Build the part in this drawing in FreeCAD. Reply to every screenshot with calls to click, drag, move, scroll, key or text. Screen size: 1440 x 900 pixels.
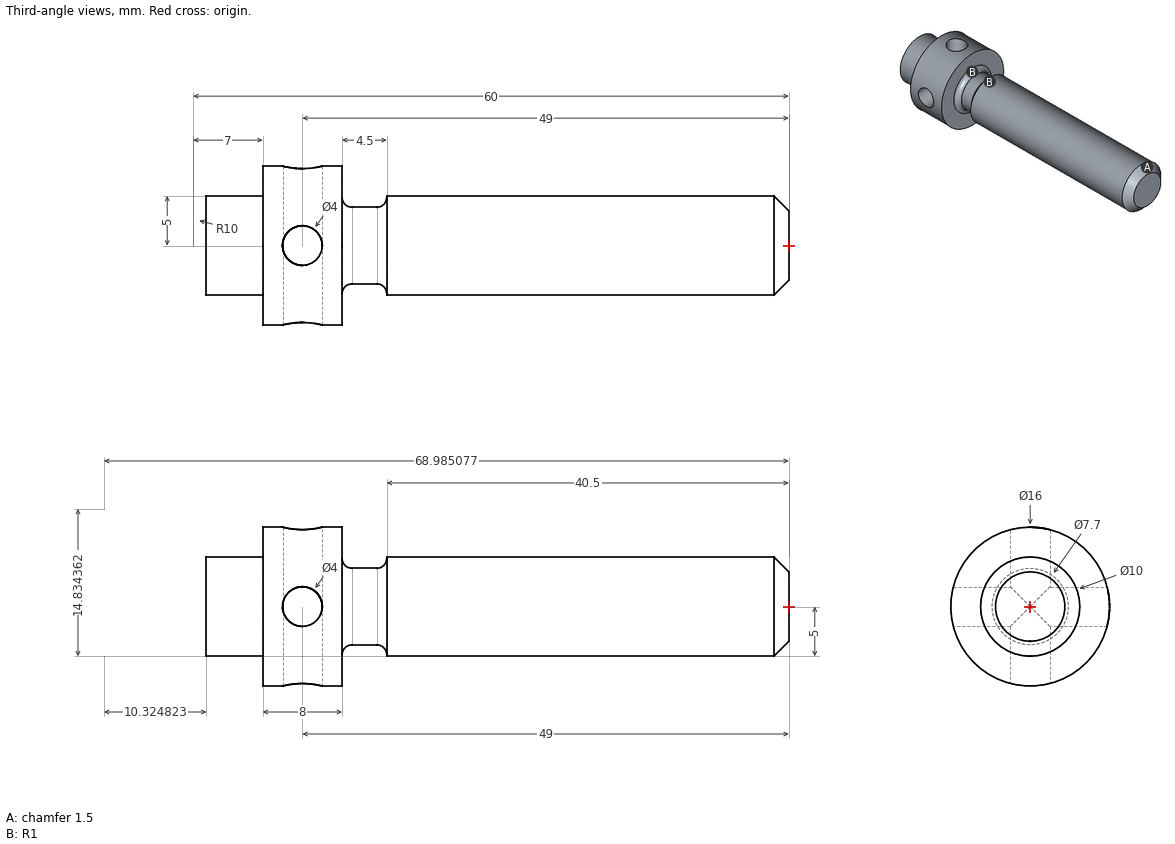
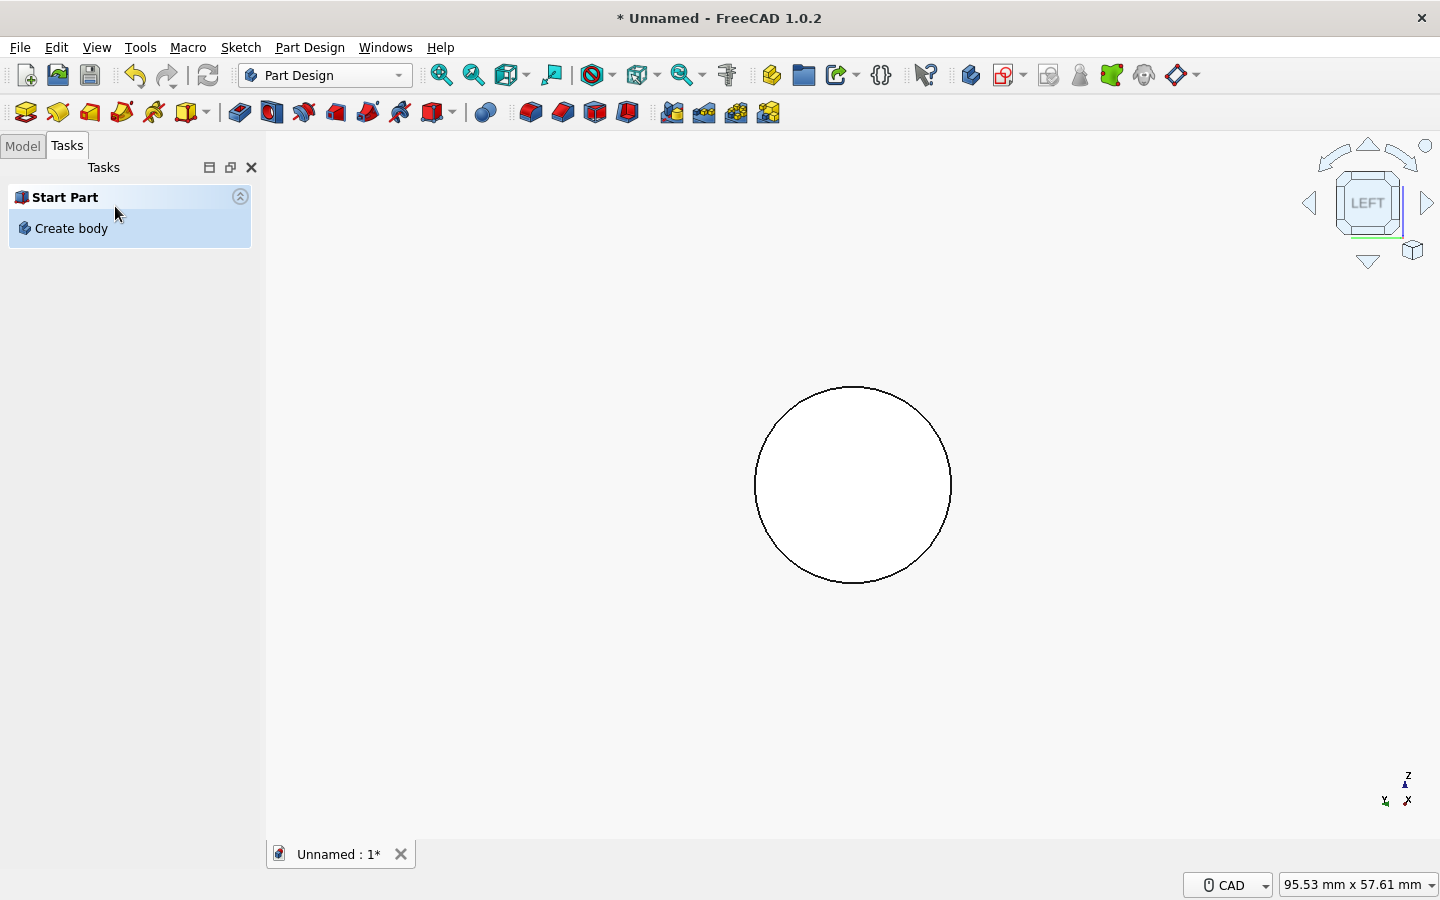
click(1004, 76)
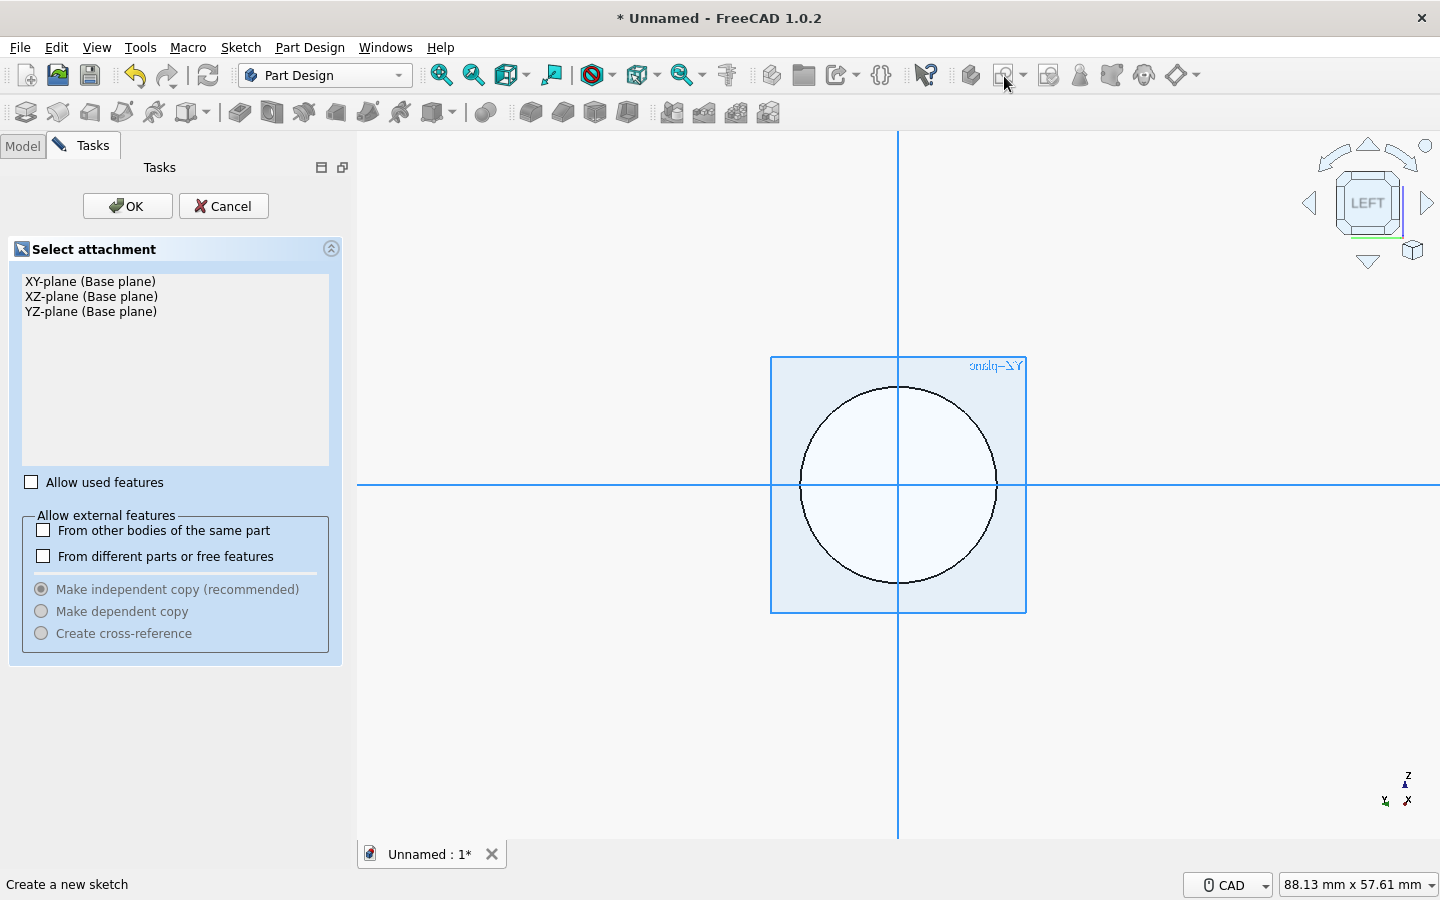
click(82, 282)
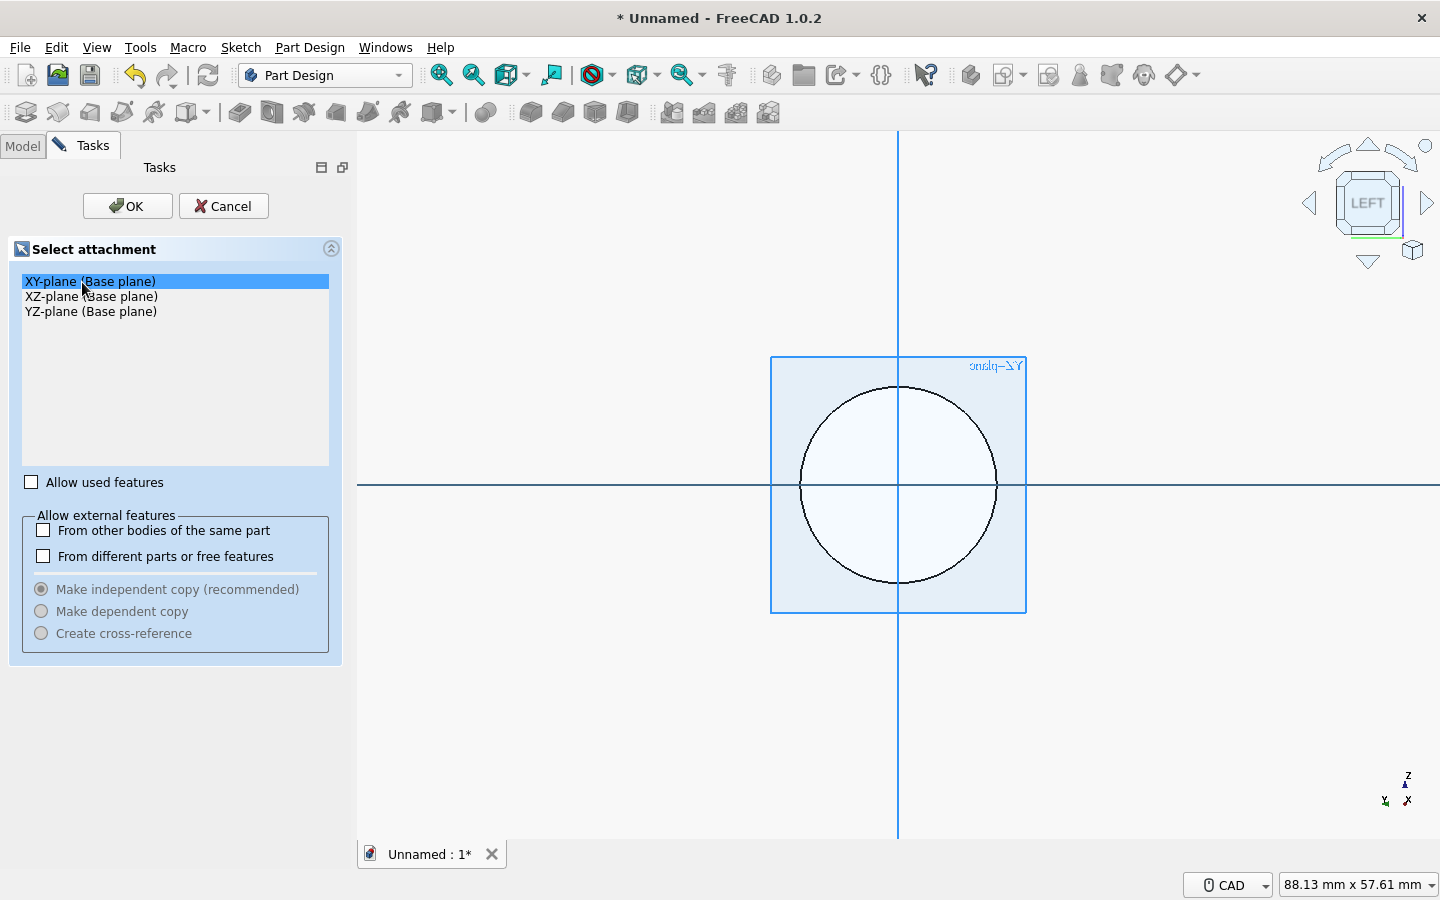
click(128, 206)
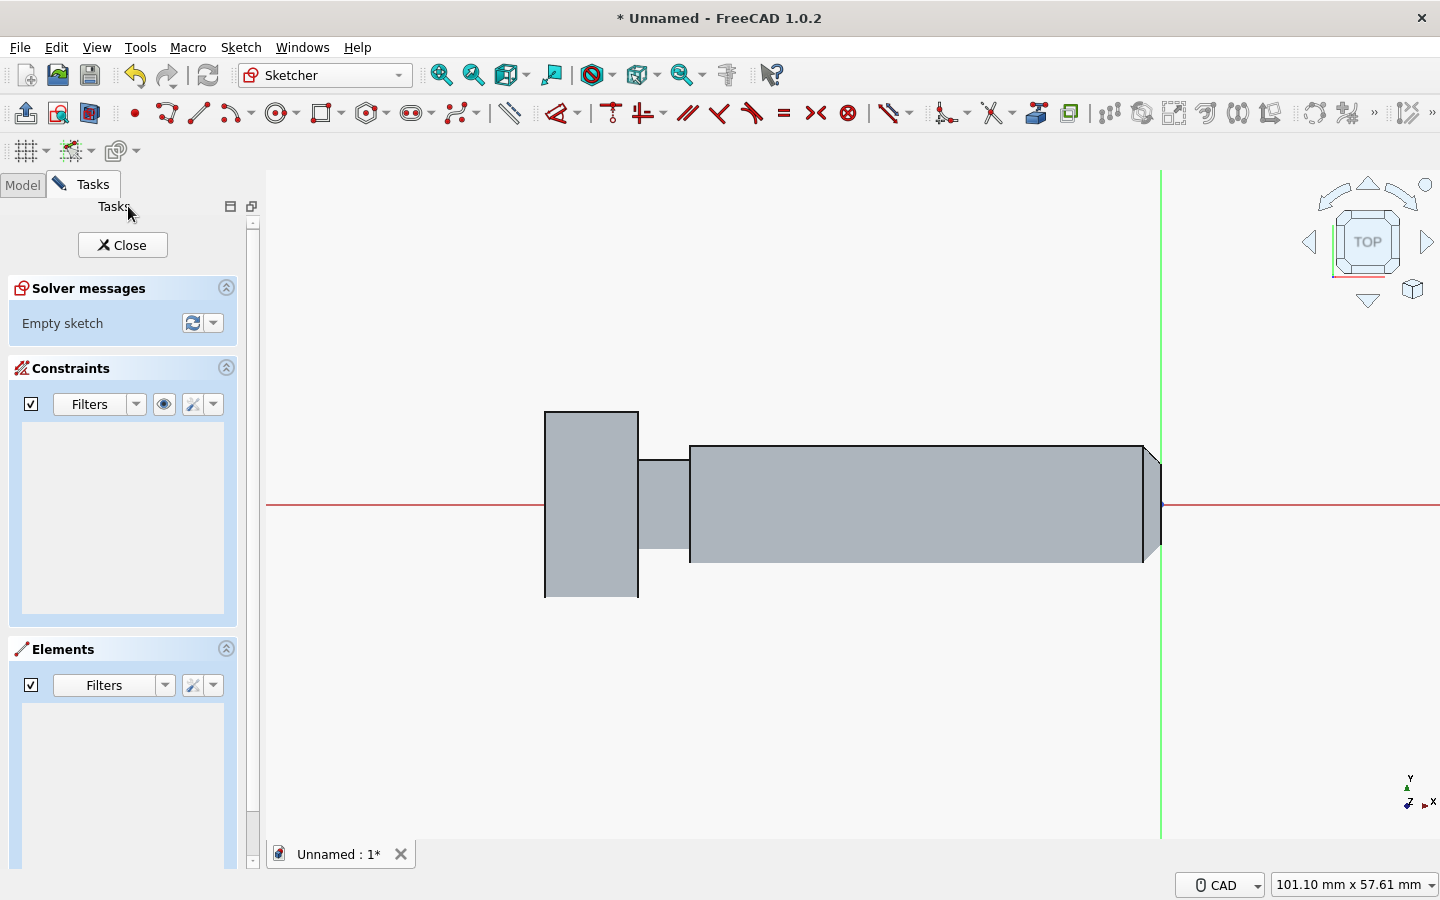
key(q)
key(s)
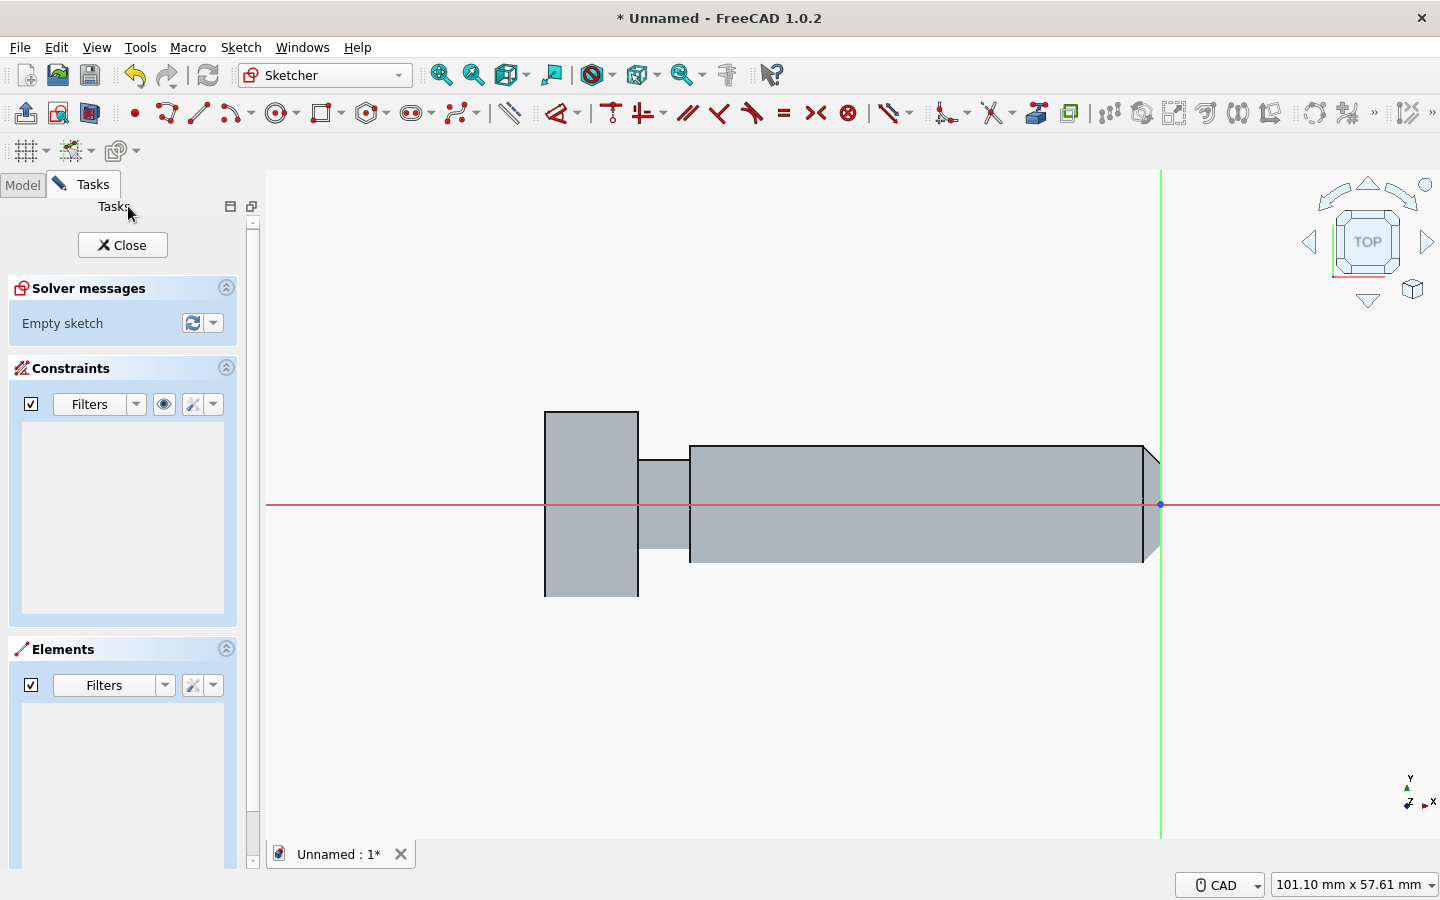
scroll(568, 504, up, 11)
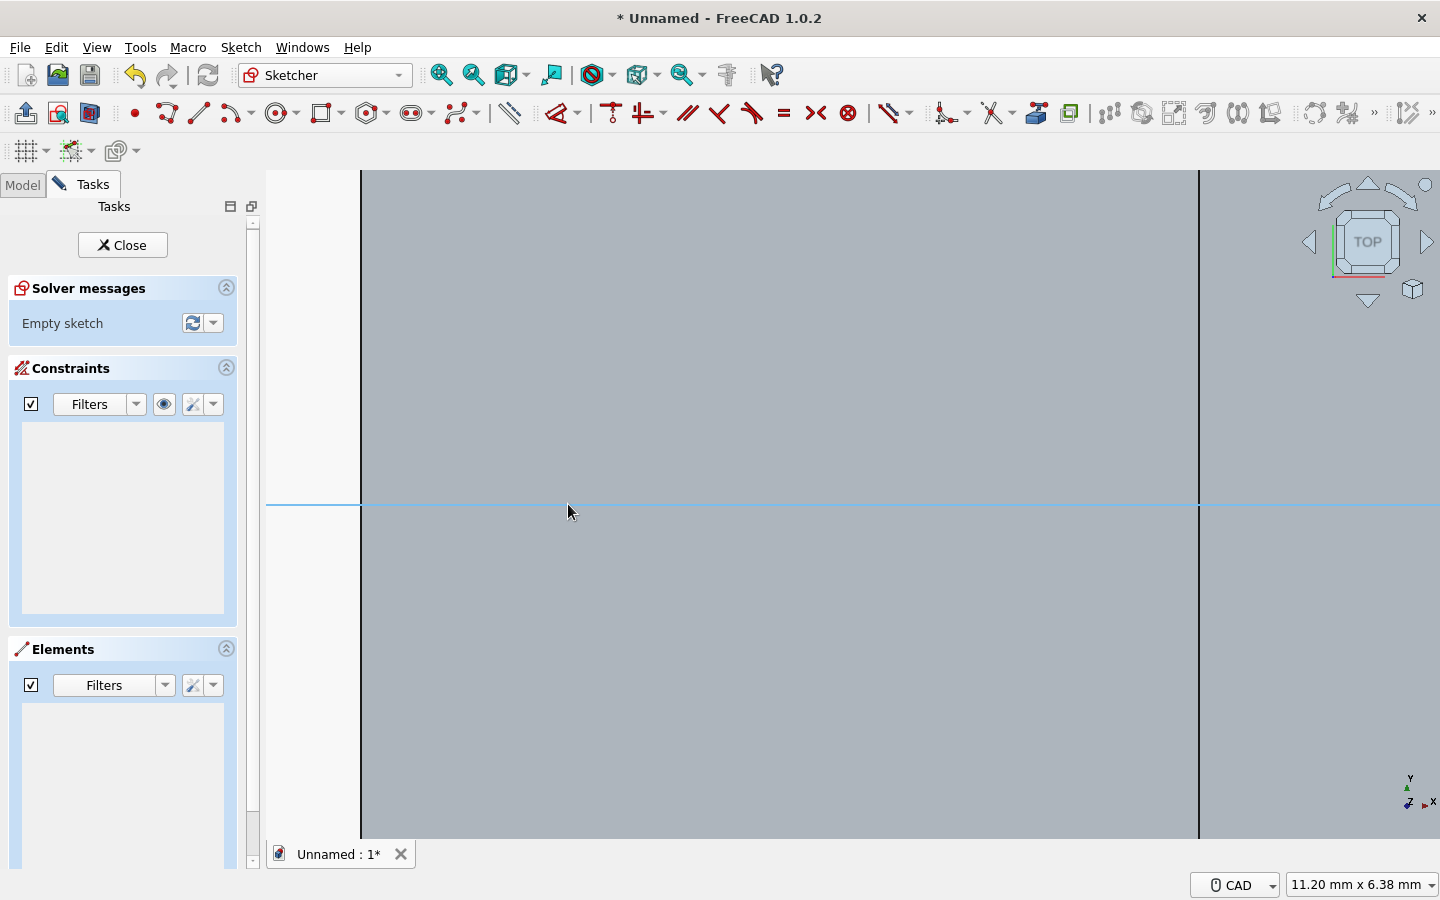
click(276, 114)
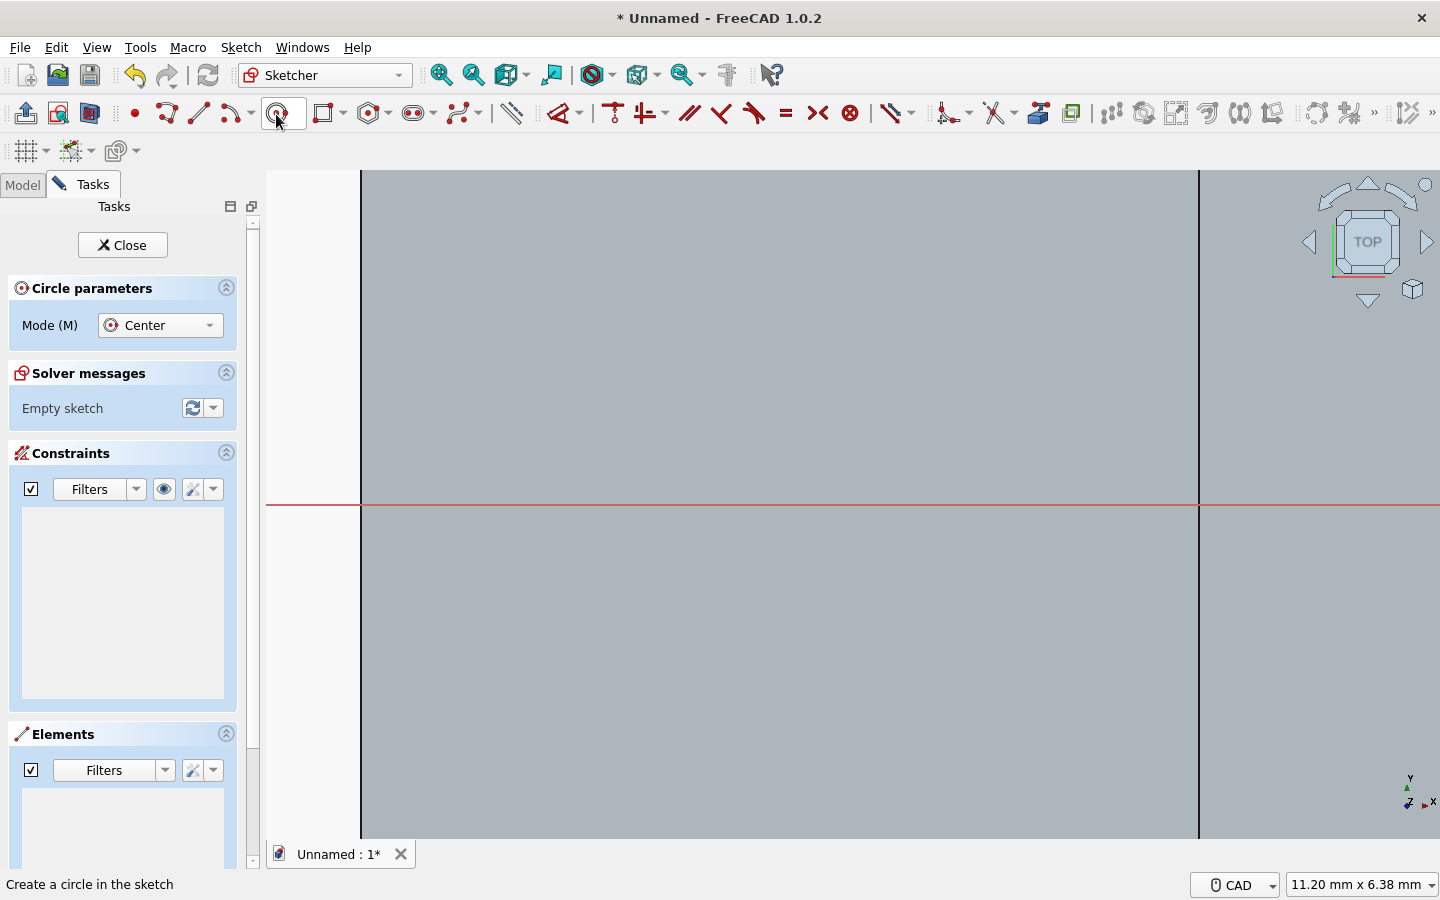
click(780, 504)
click(928, 356)
key(Escape)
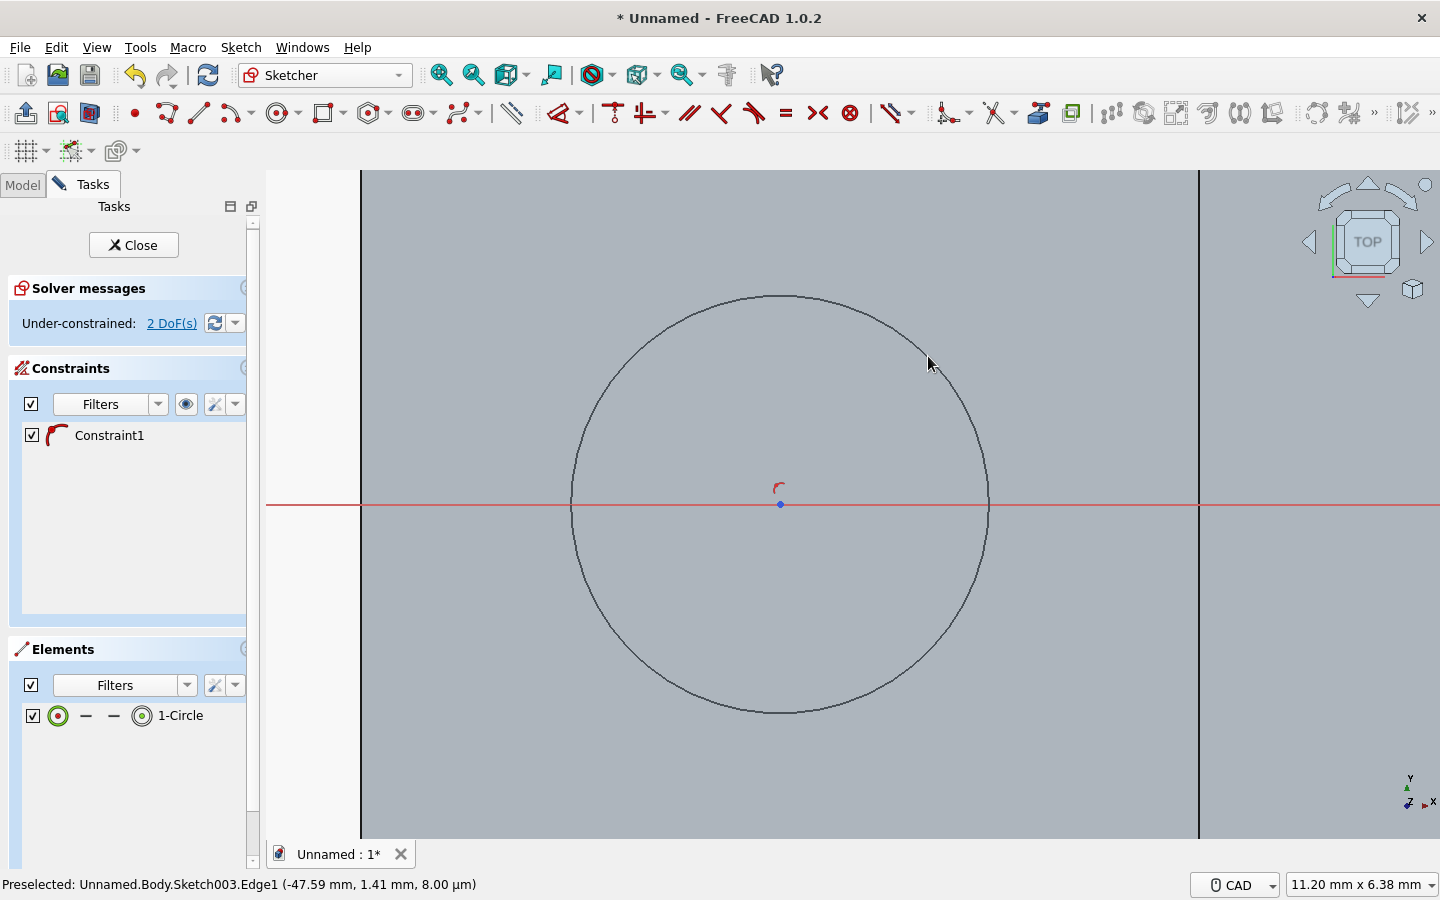
key(d)